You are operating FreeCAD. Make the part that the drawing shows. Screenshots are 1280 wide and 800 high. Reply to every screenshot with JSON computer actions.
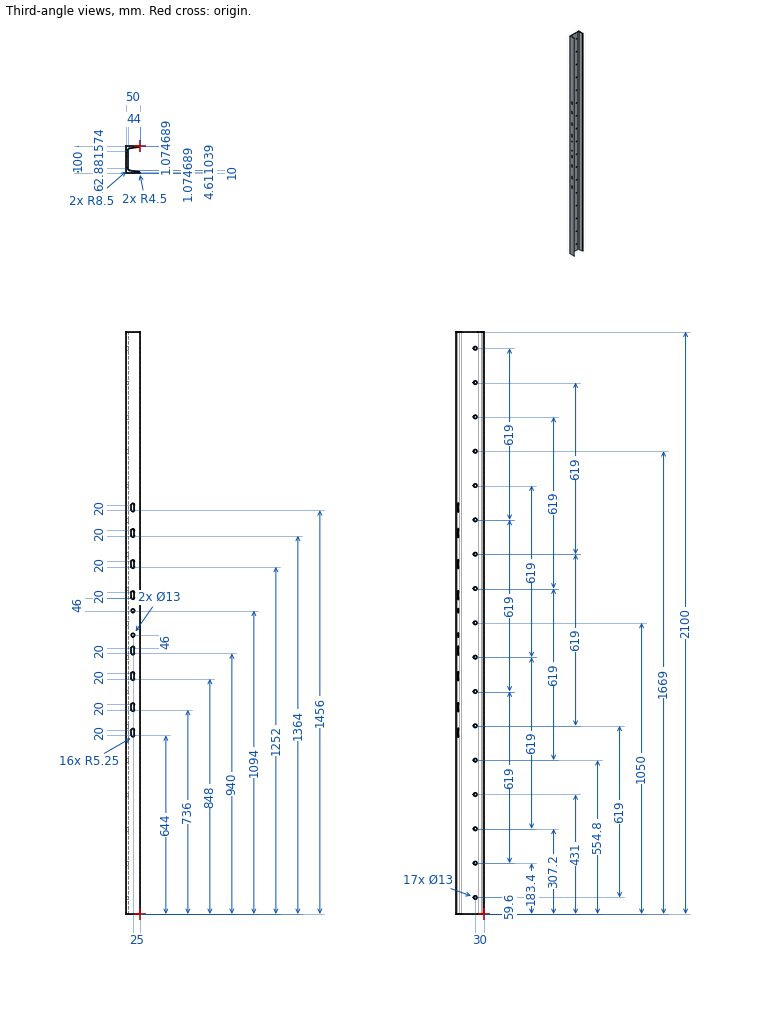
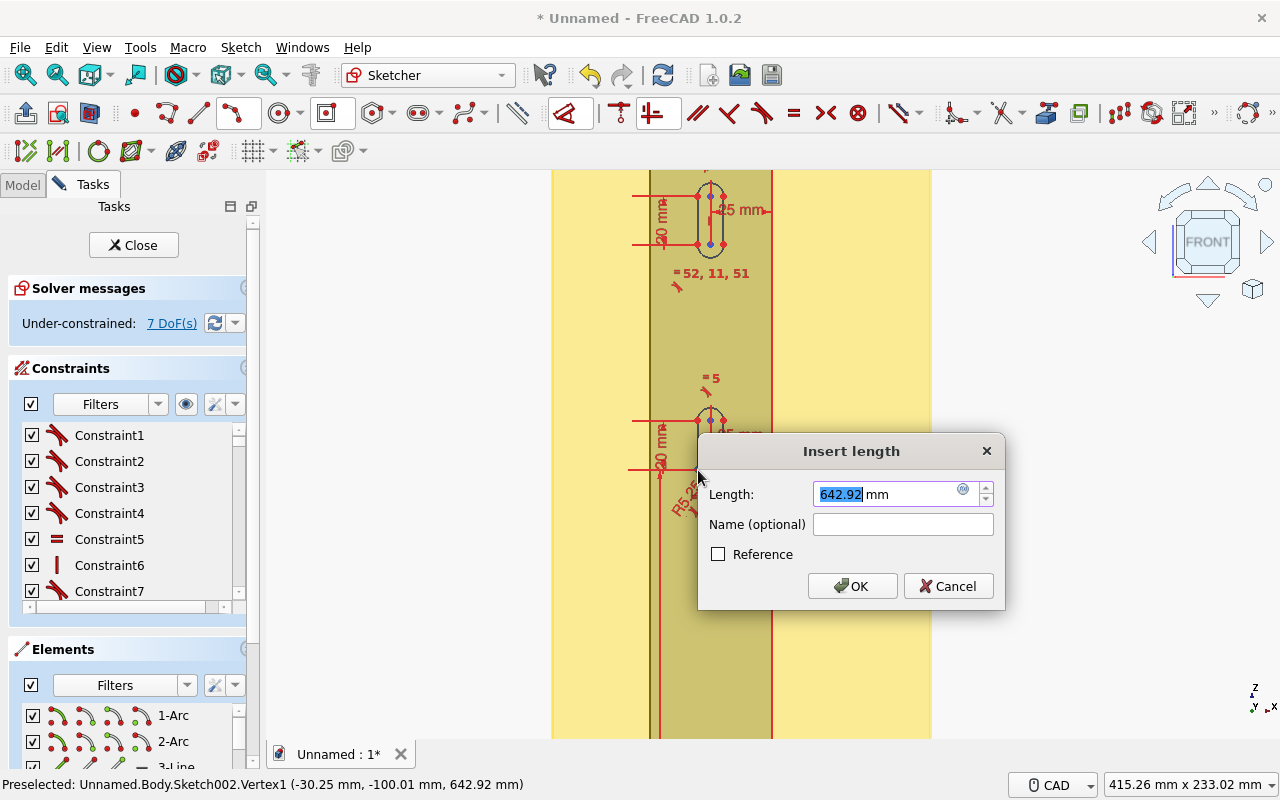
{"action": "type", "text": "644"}
{"action": "key", "text": "Return"}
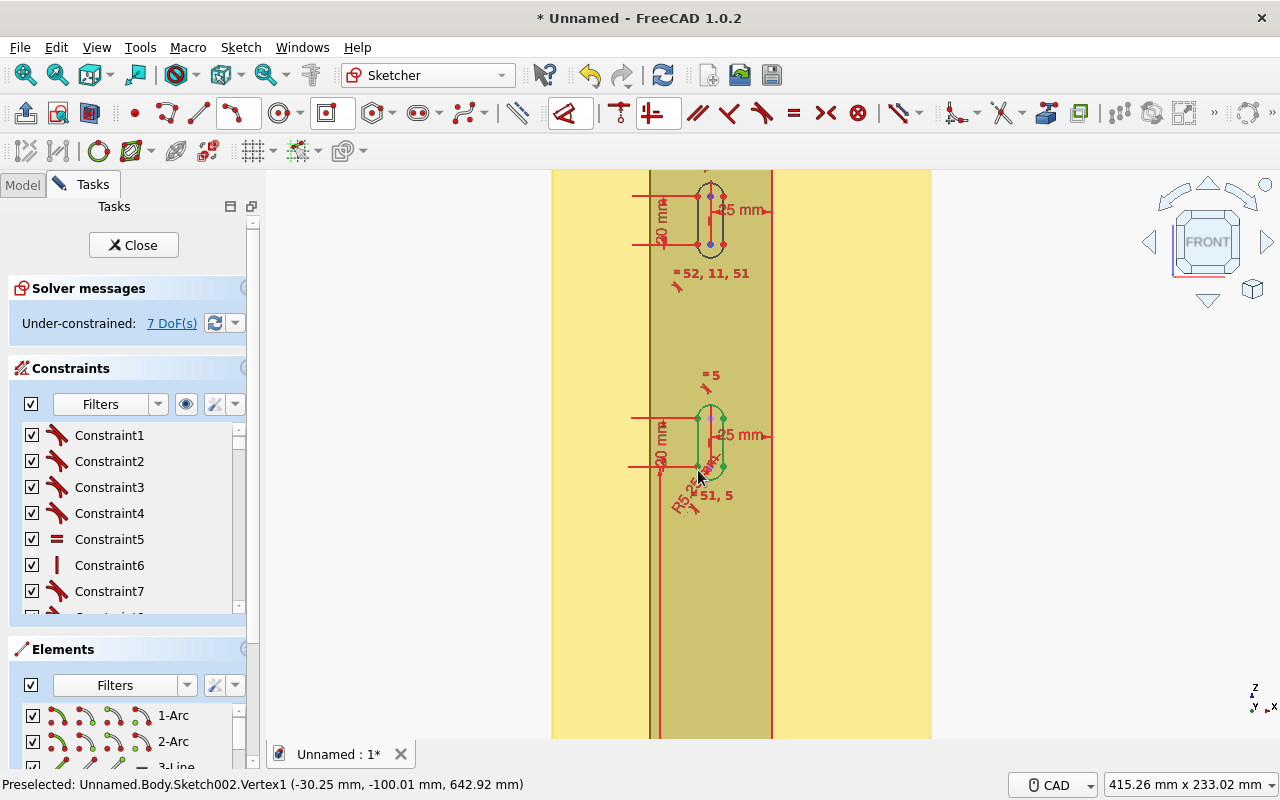
{"action": "left_click", "coordinate": [698, 245]}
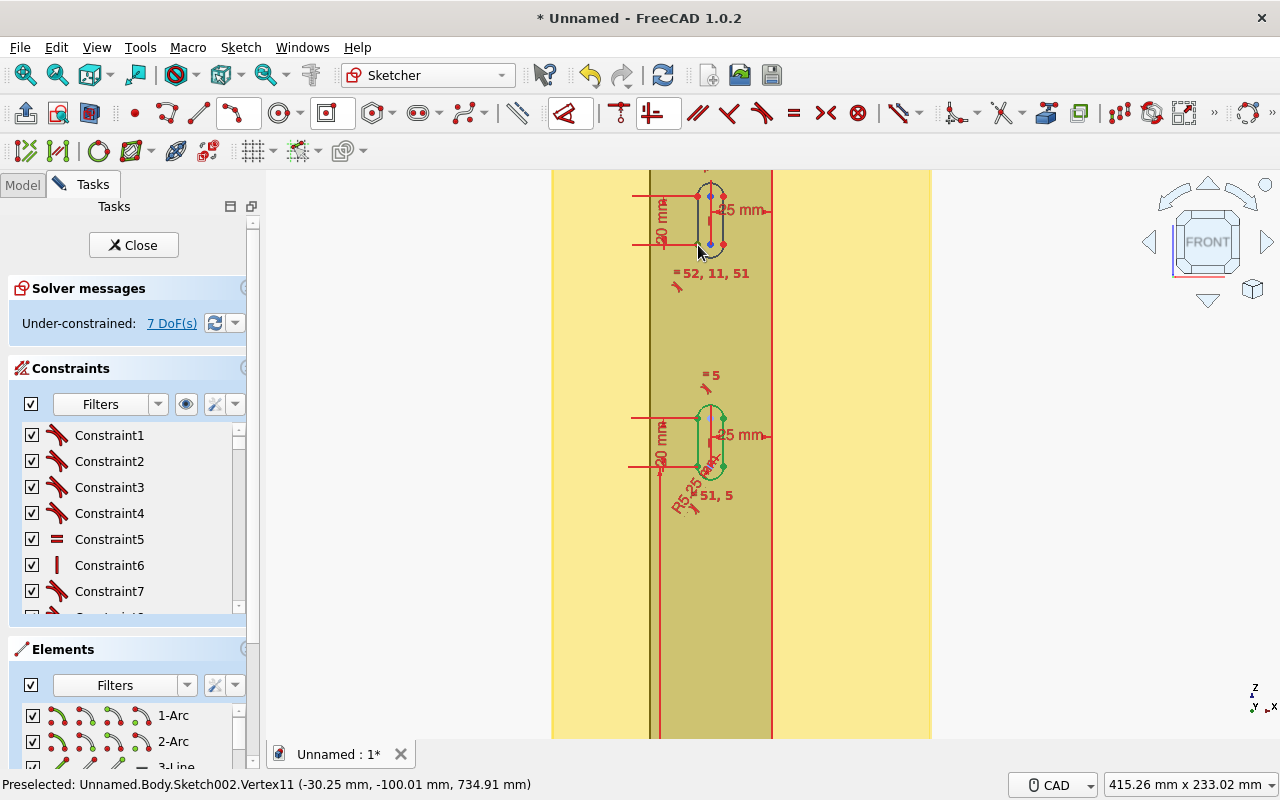
{"action": "key", "text": "i"}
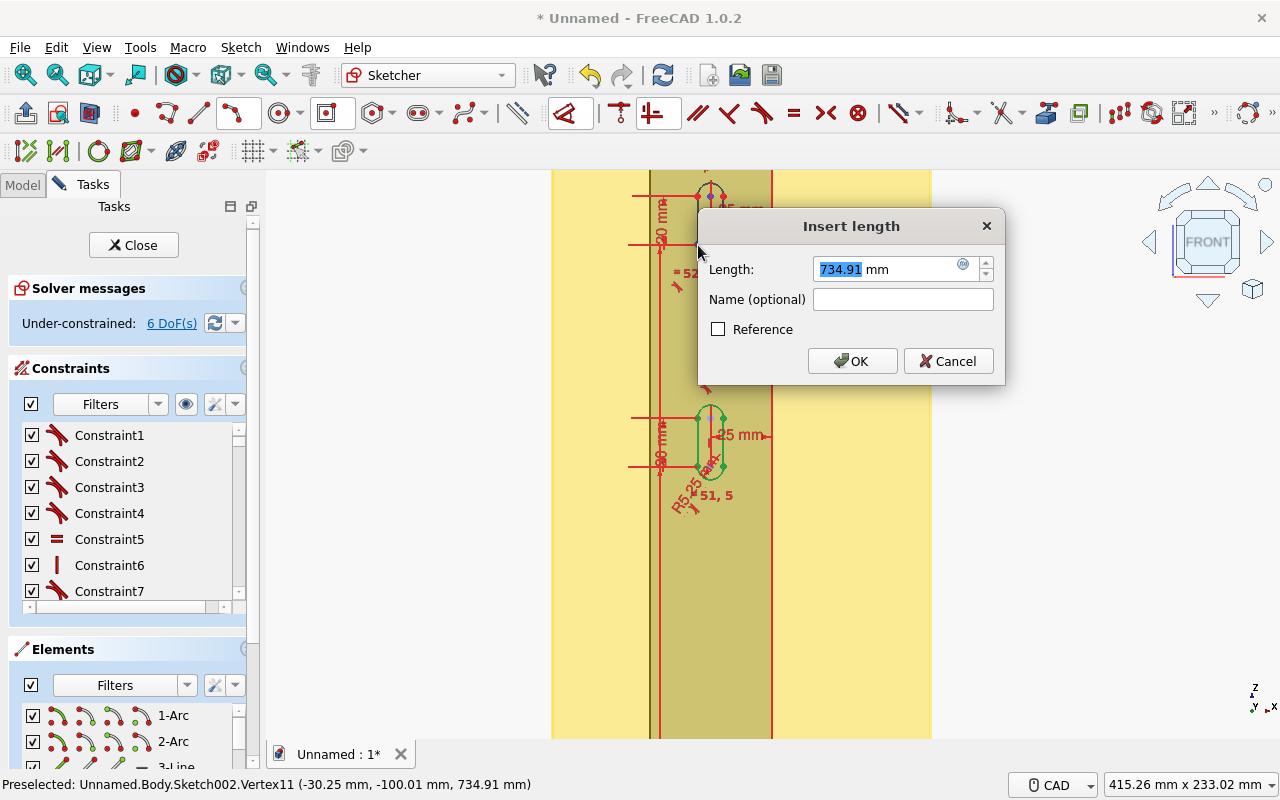
{"action": "type", "text": "736"}
{"action": "key", "text": "Return"}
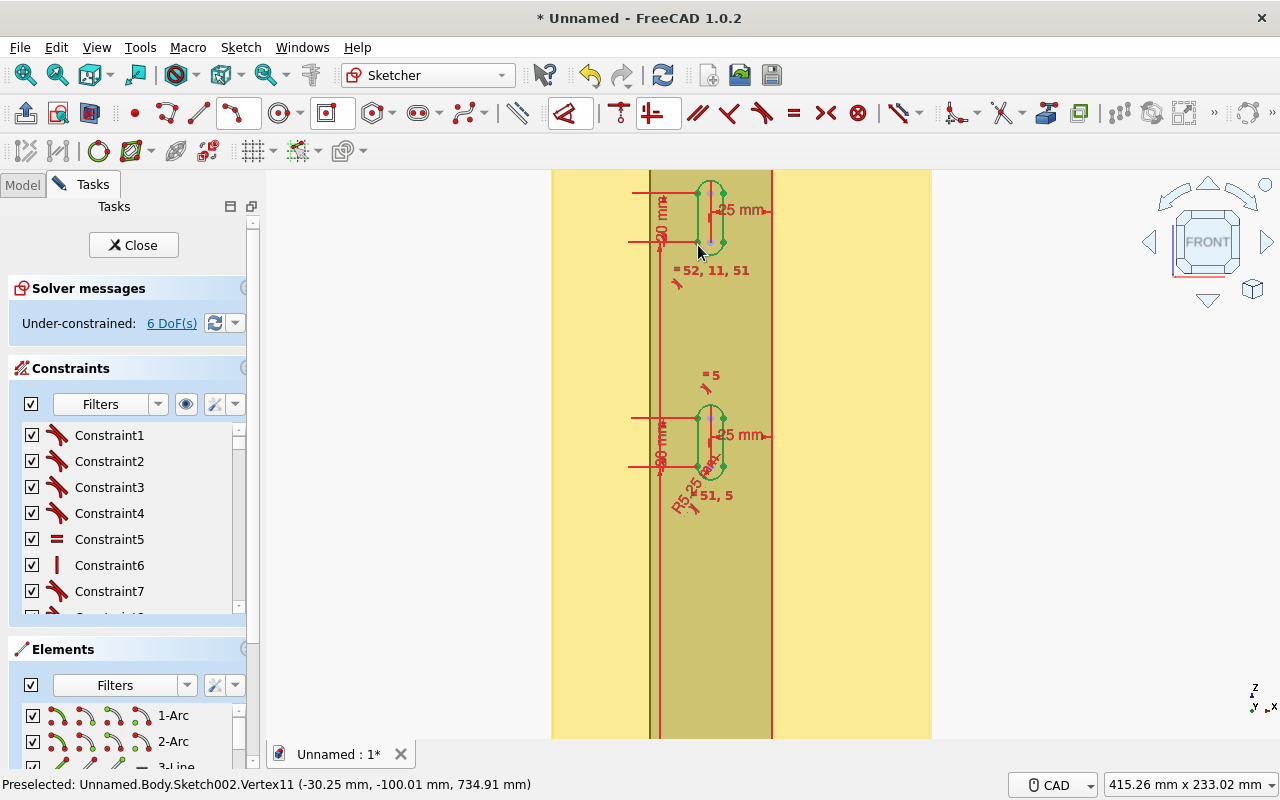
{"action": "scroll", "coordinate": [702, 477], "scroll_direction": "down", "scroll_amount": 12}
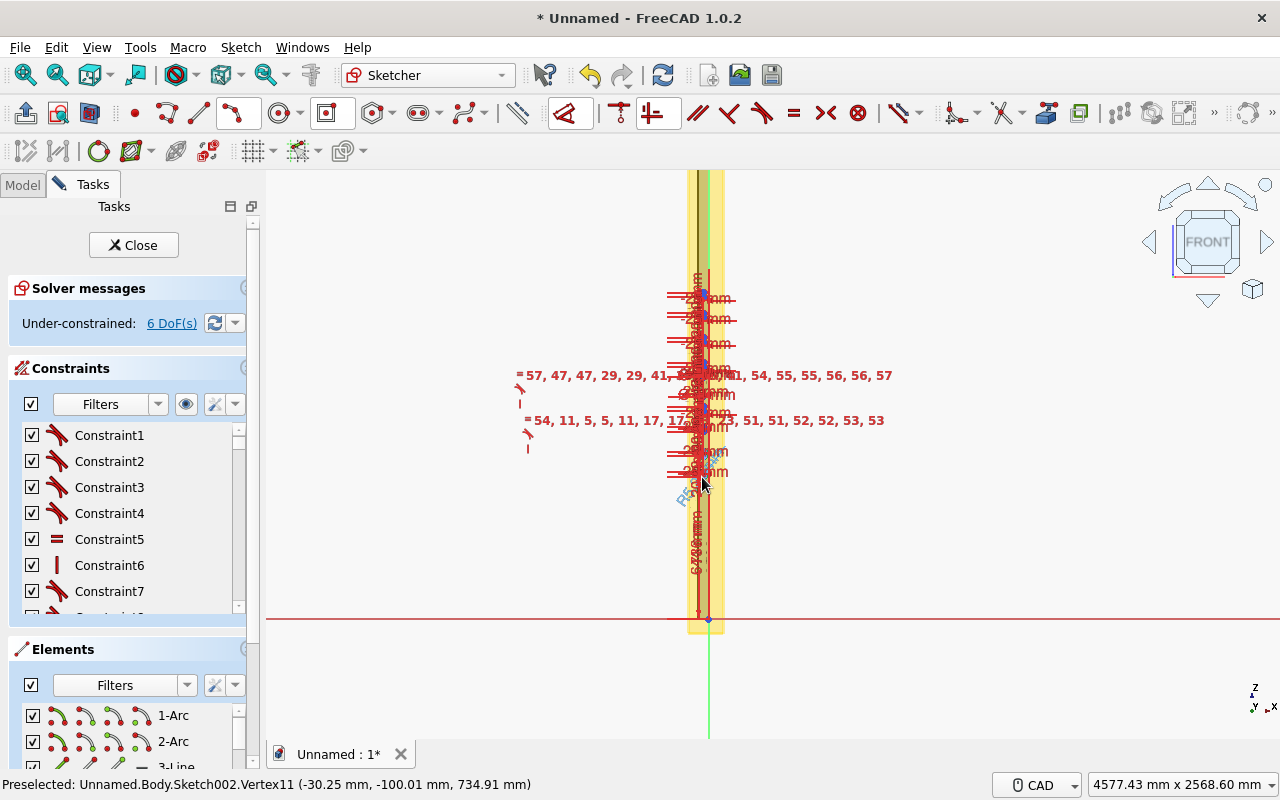
{"action": "scroll", "coordinate": [702, 432], "scroll_direction": "up", "scroll_amount": 12}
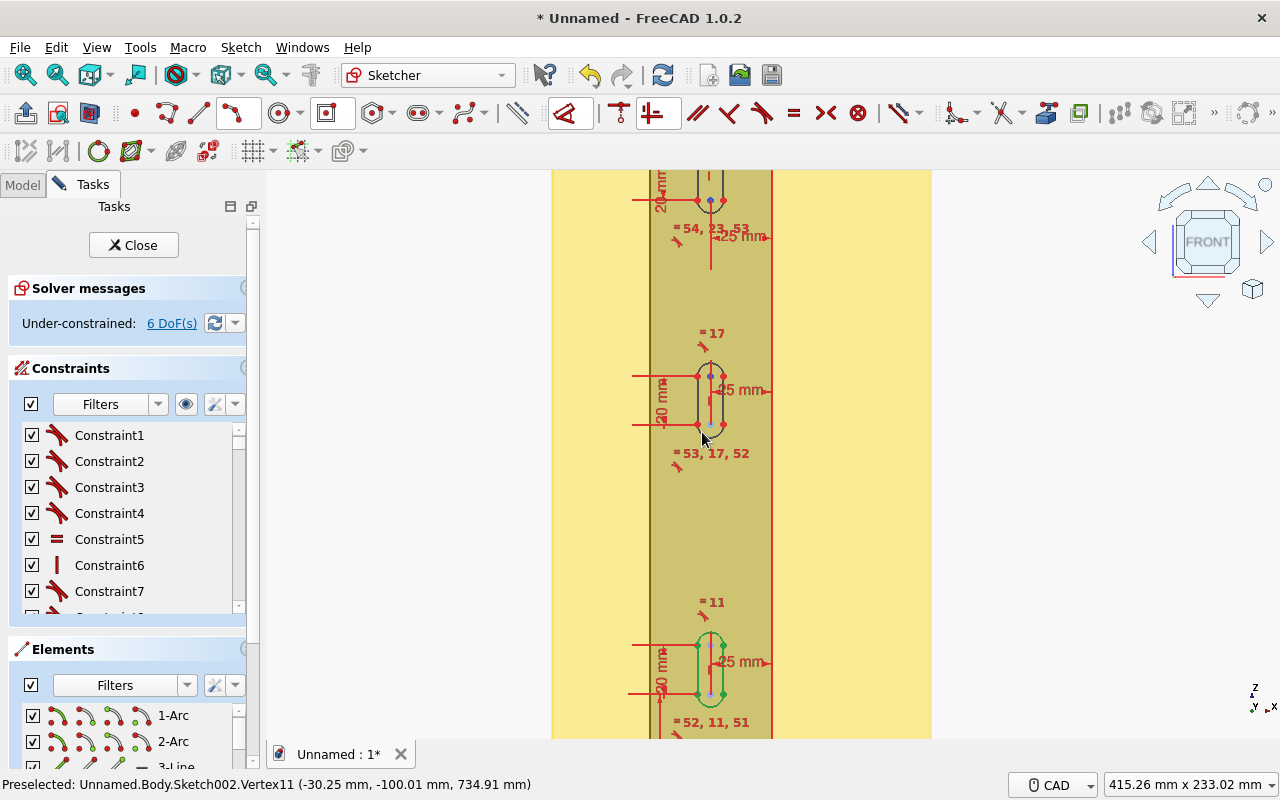
{"action": "left_click", "coordinate": [698, 425]}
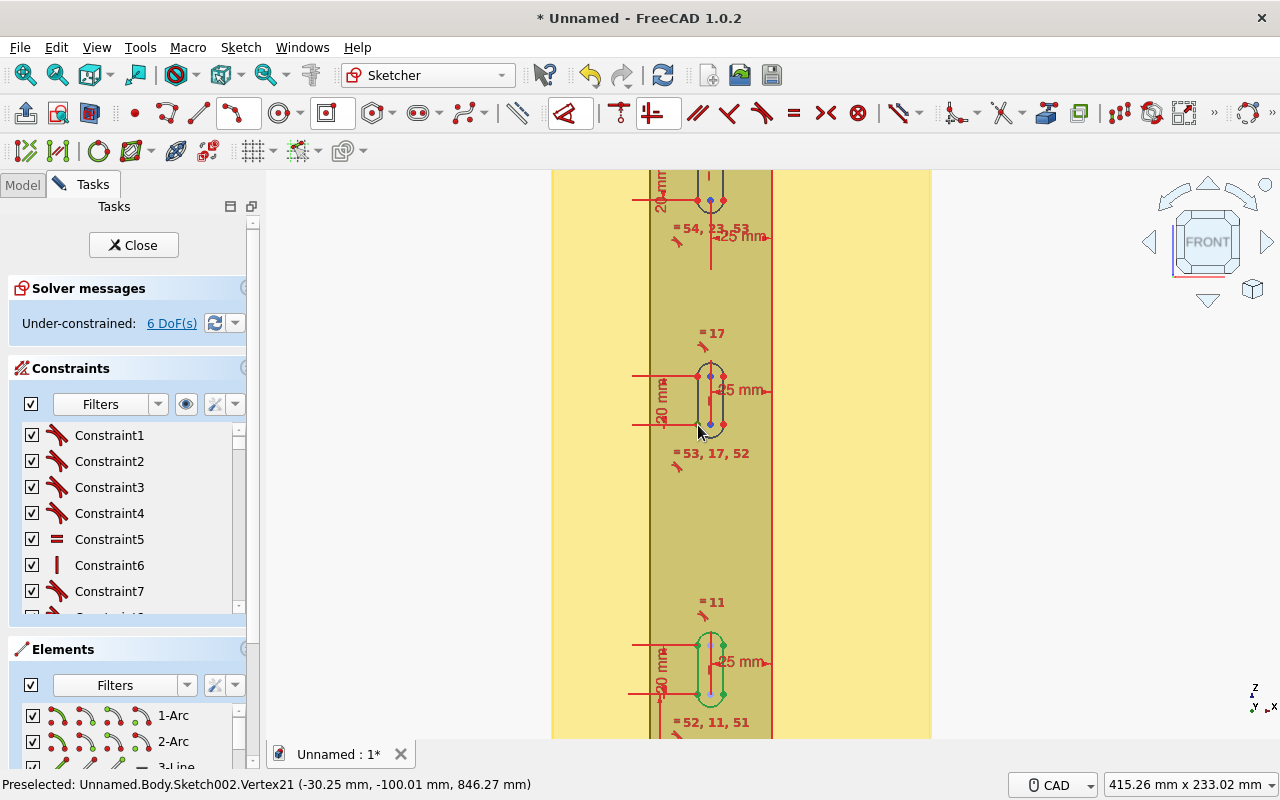
{"action": "key", "text": "i"}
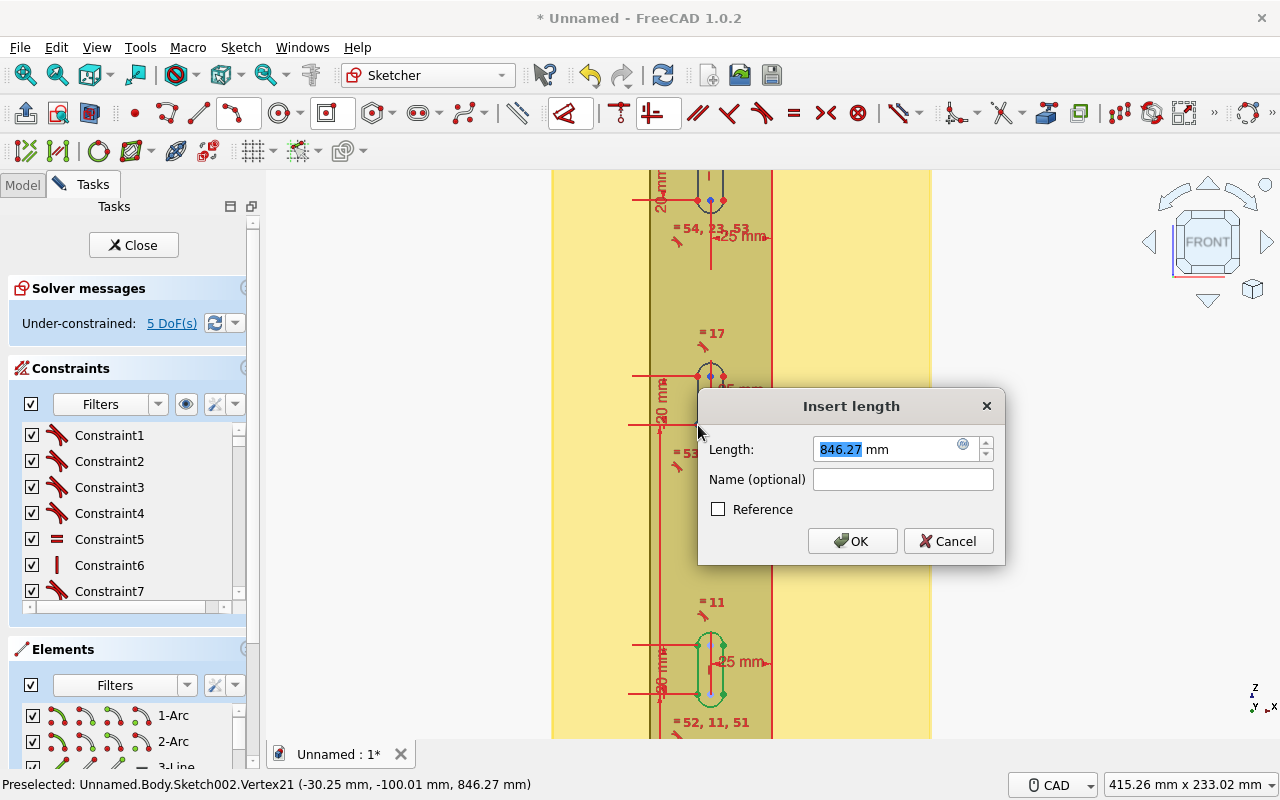
{"action": "type", "text": "848"}
{"action": "key", "text": "Return"}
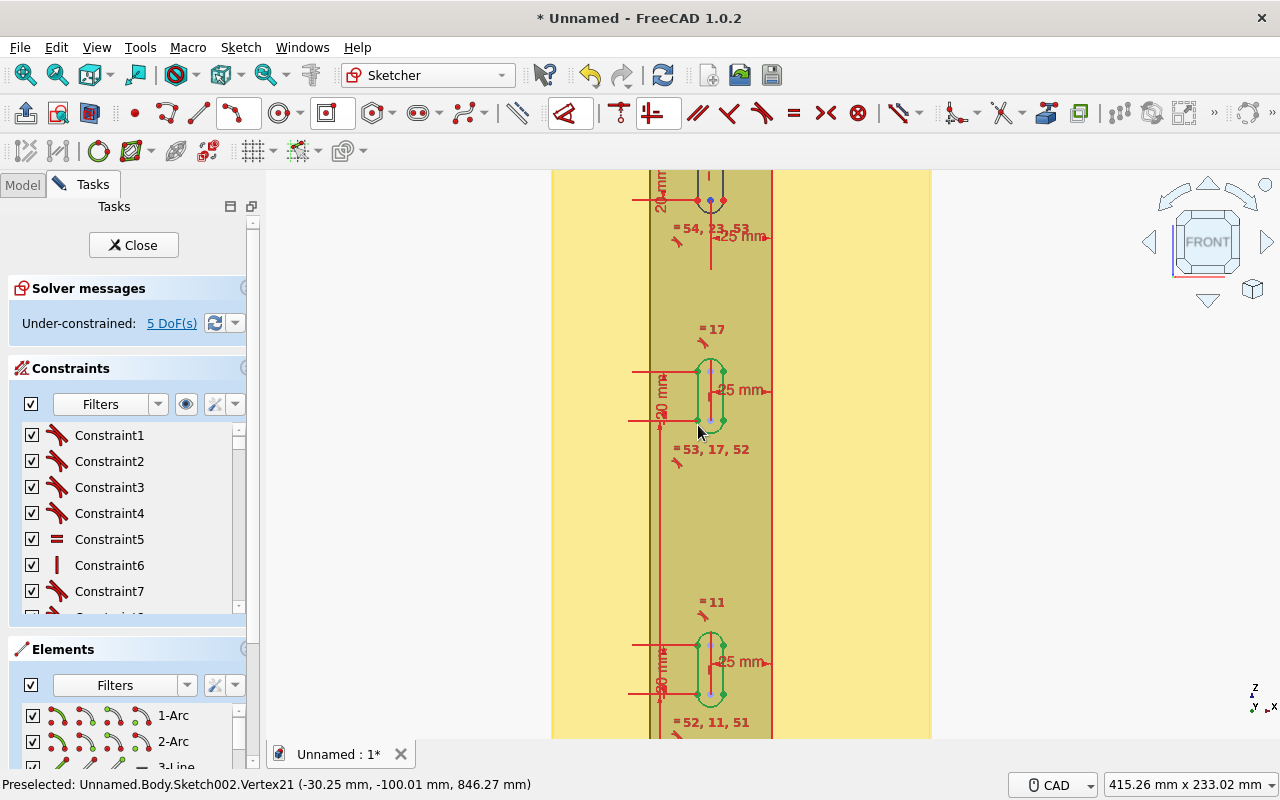
{"action": "left_click", "coordinate": [698, 200]}